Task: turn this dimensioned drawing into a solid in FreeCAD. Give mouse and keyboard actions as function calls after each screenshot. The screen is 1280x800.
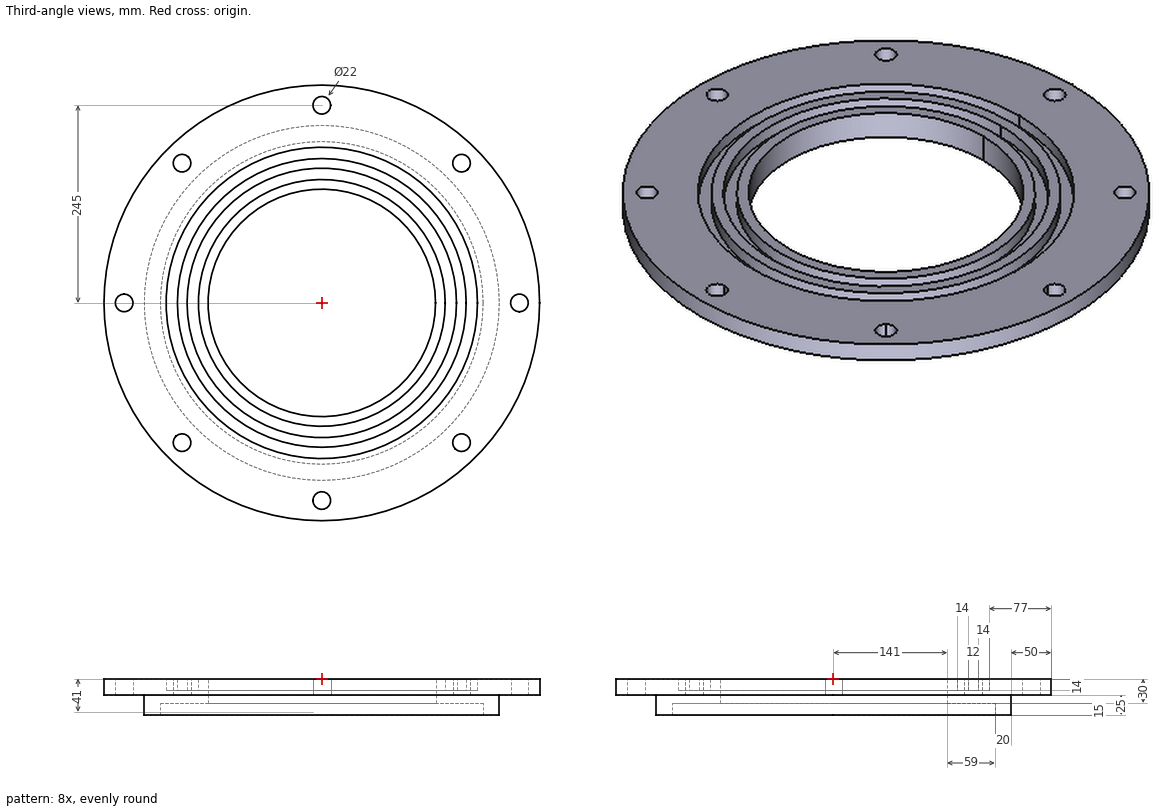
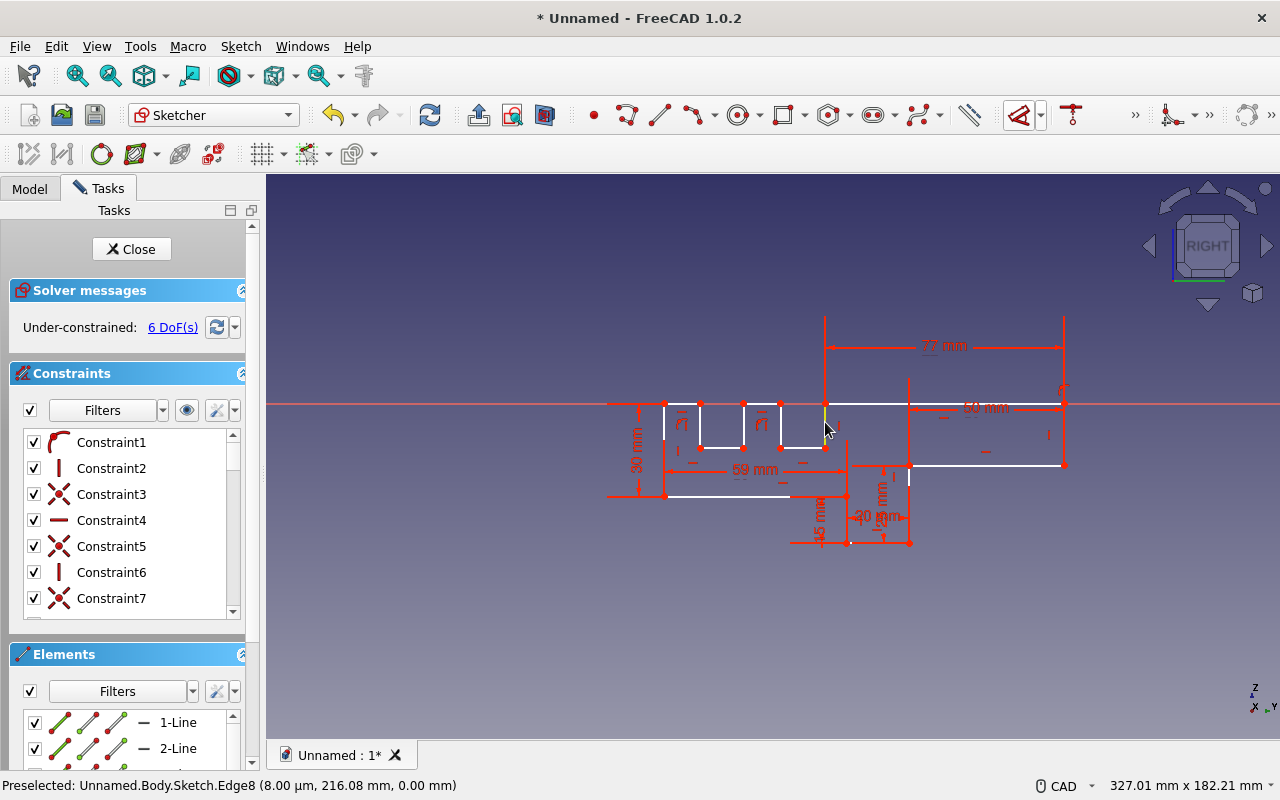
click(825, 422)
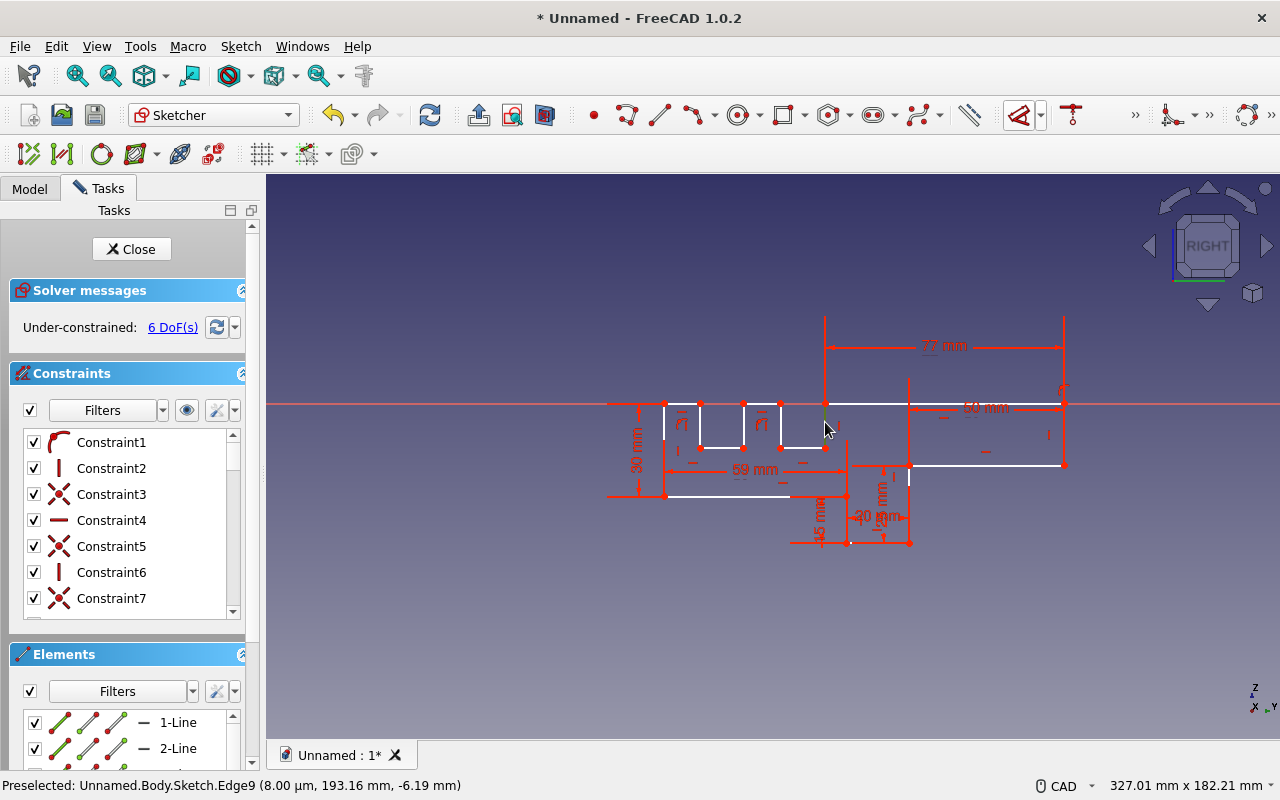
key(i)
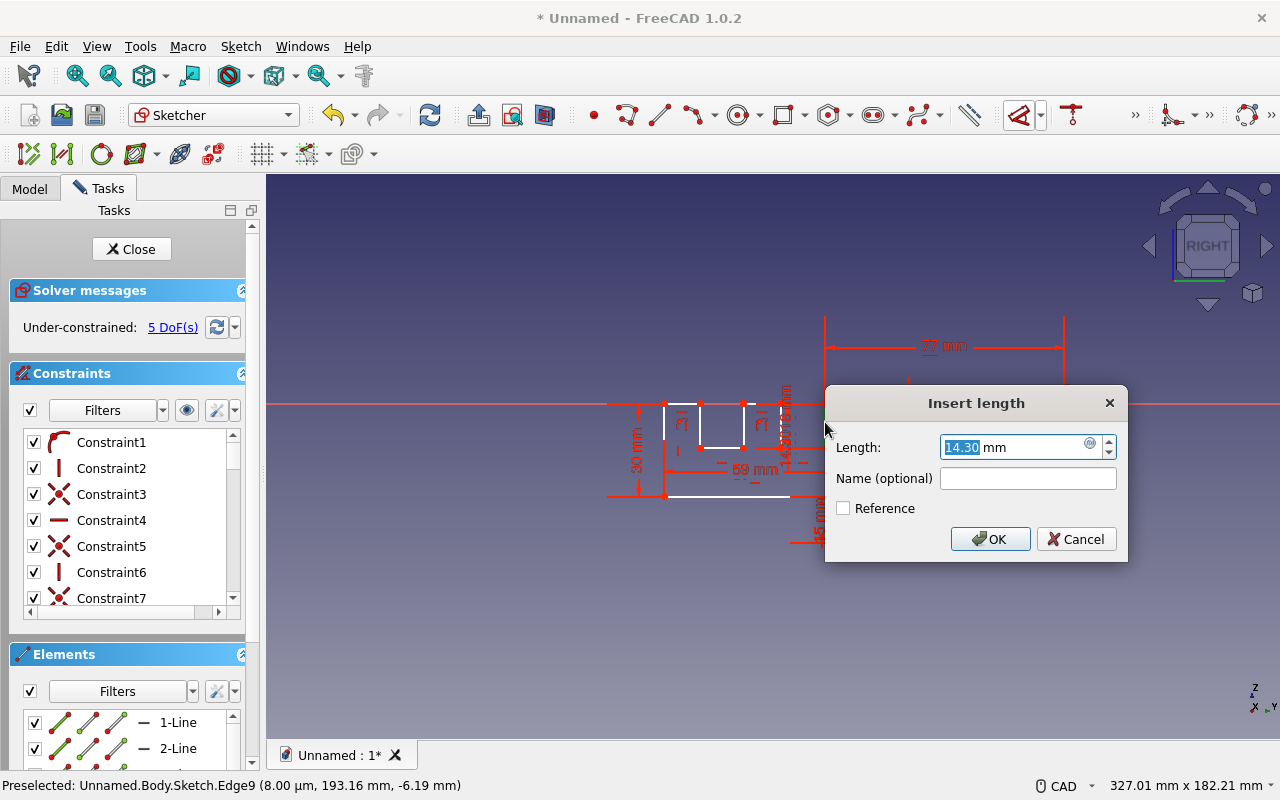
text(14)
key(Return)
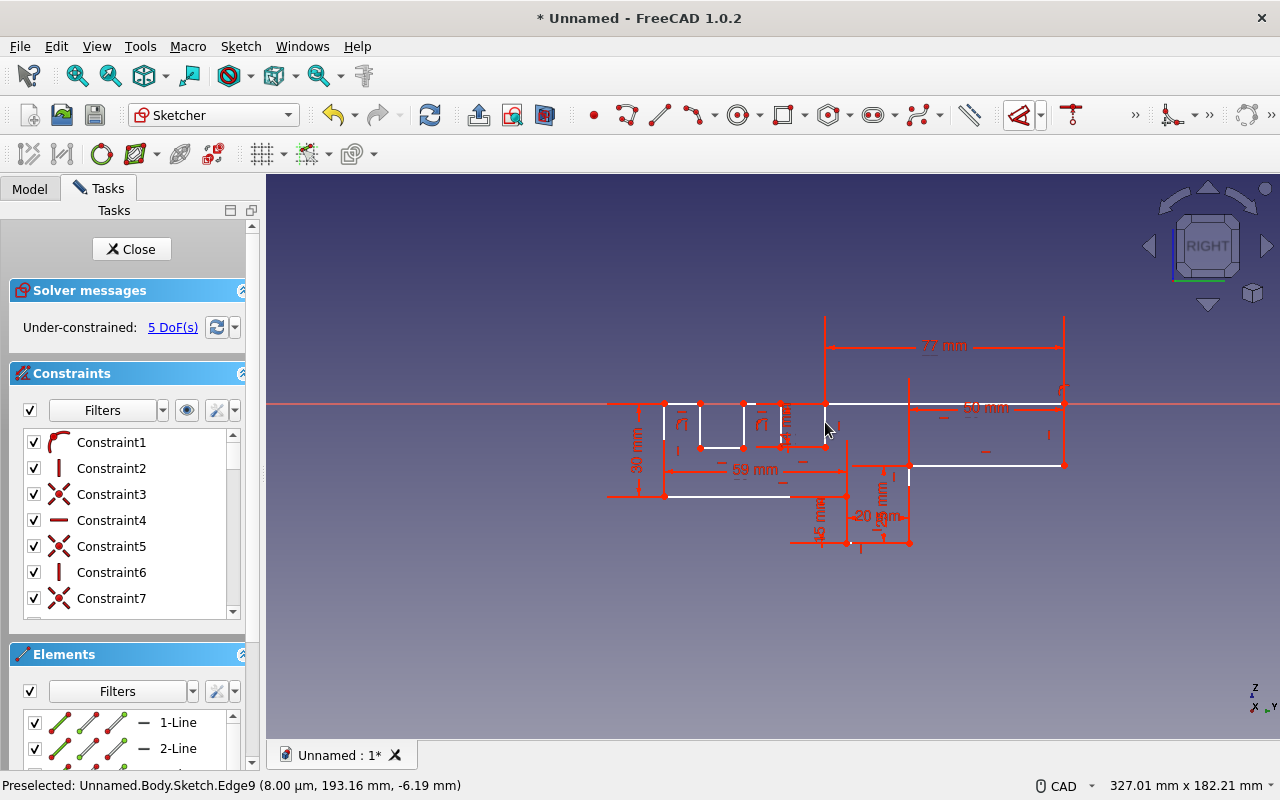
click(812, 447)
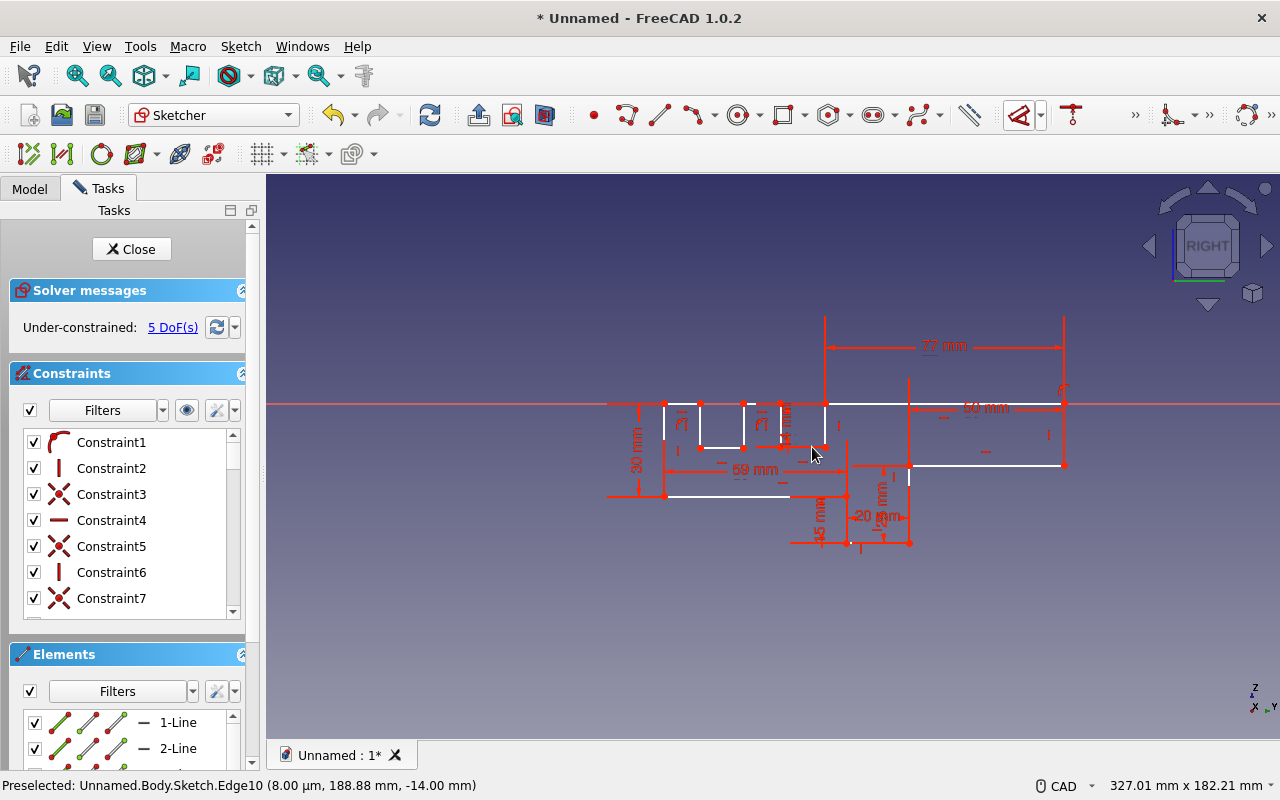
key(l)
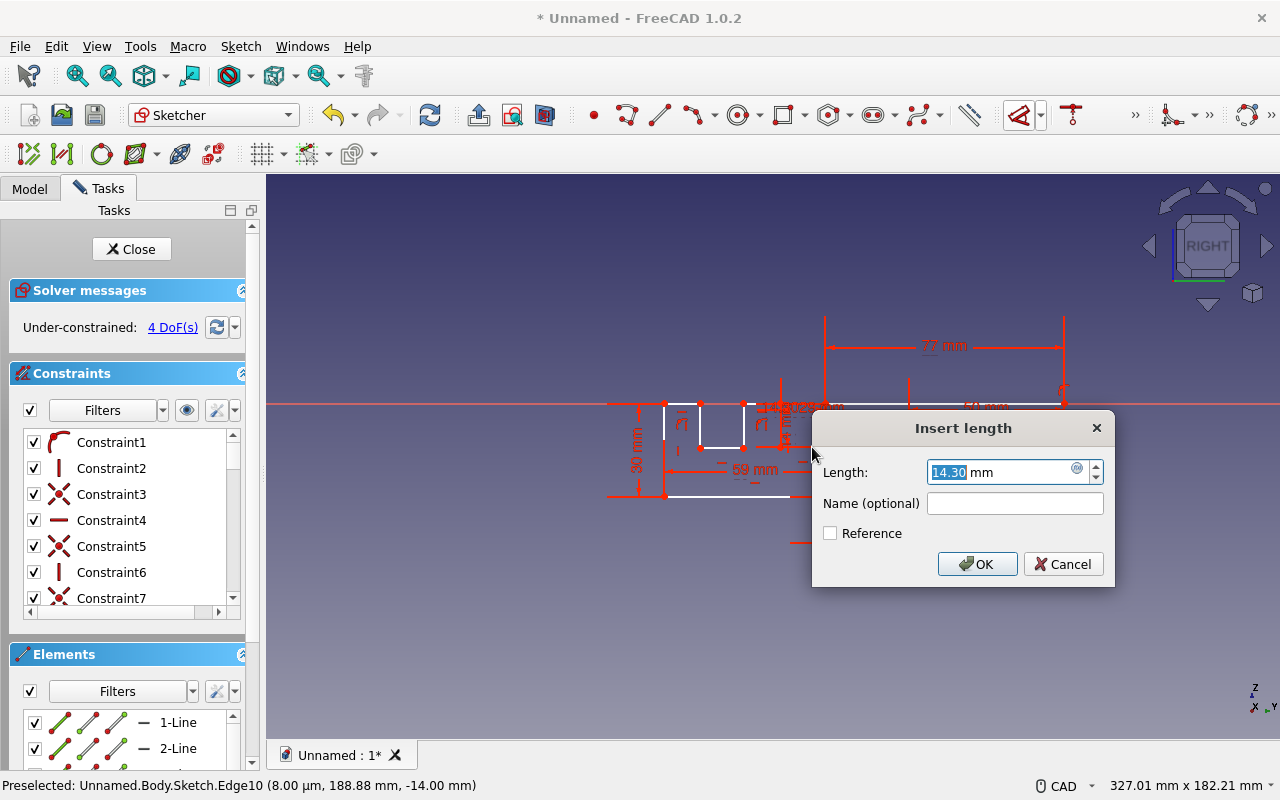
text(14)
key(Return)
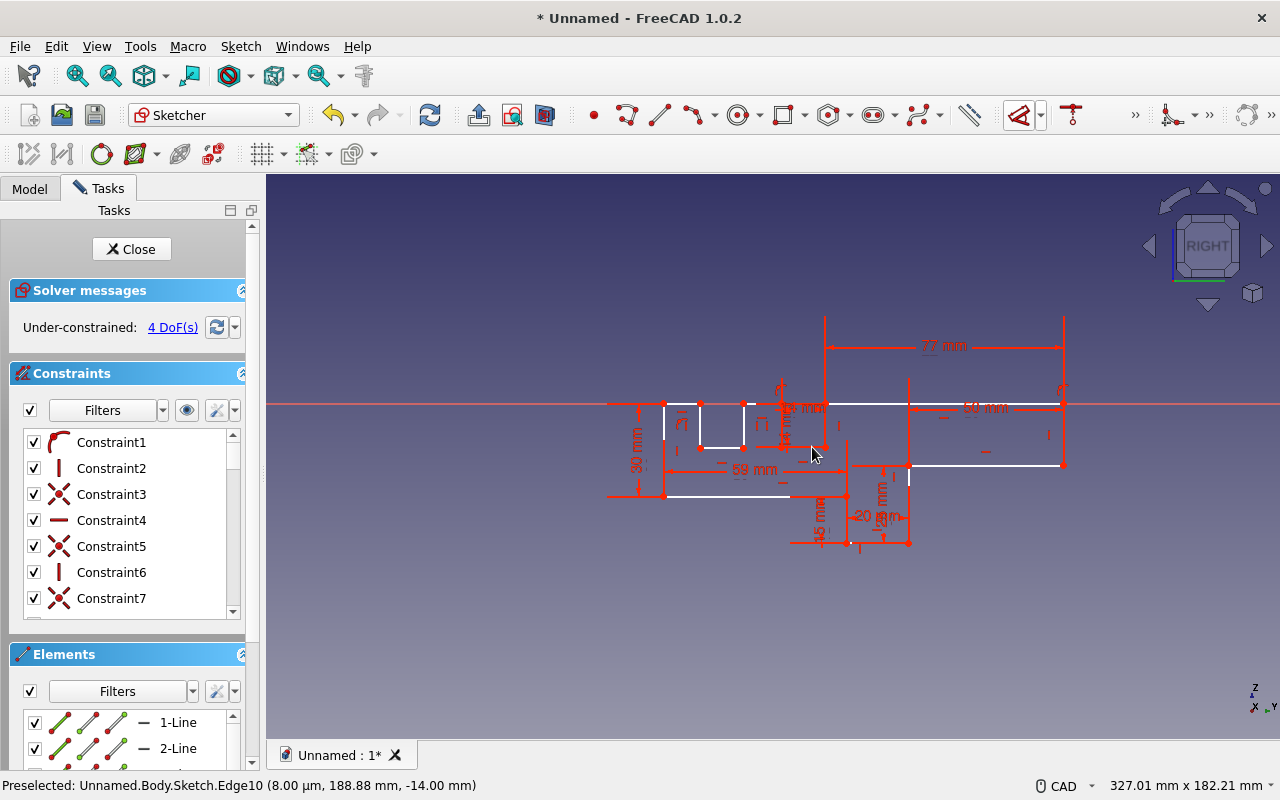
click(770, 404)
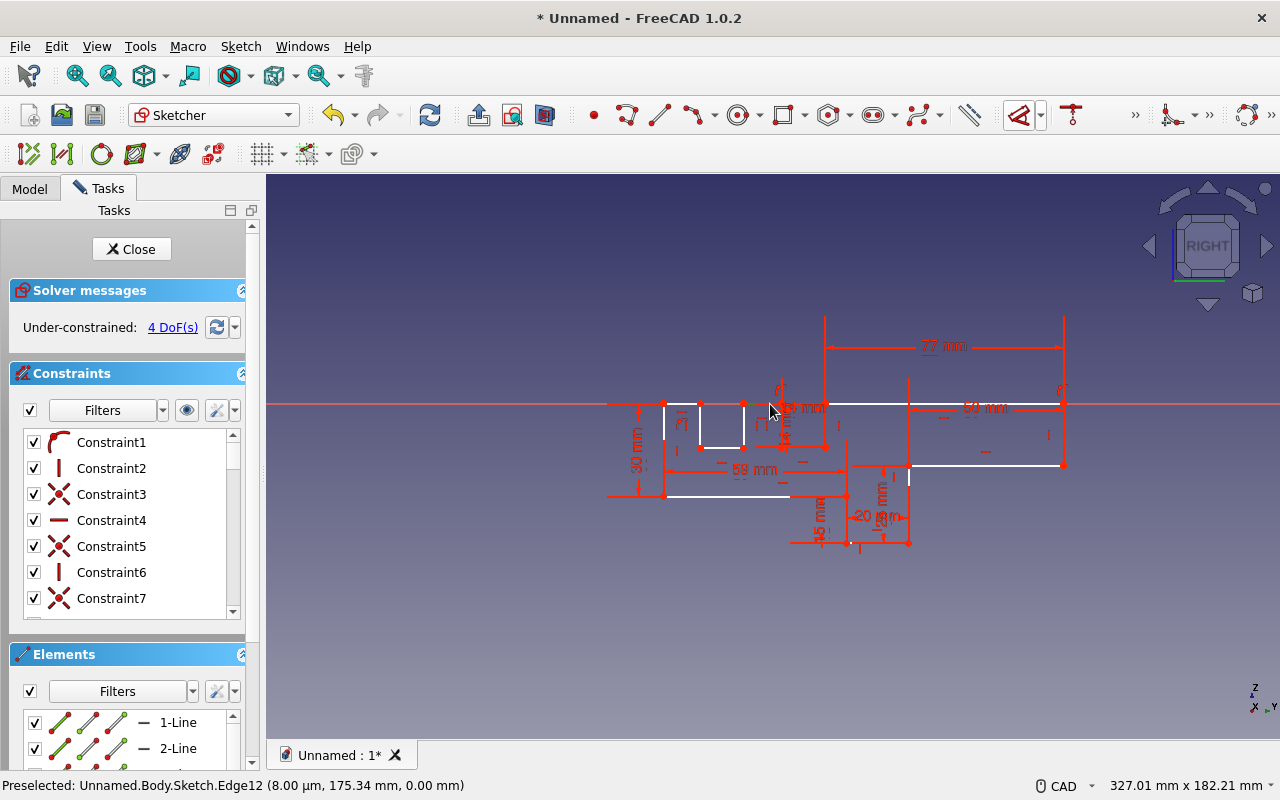
click(1040, 116)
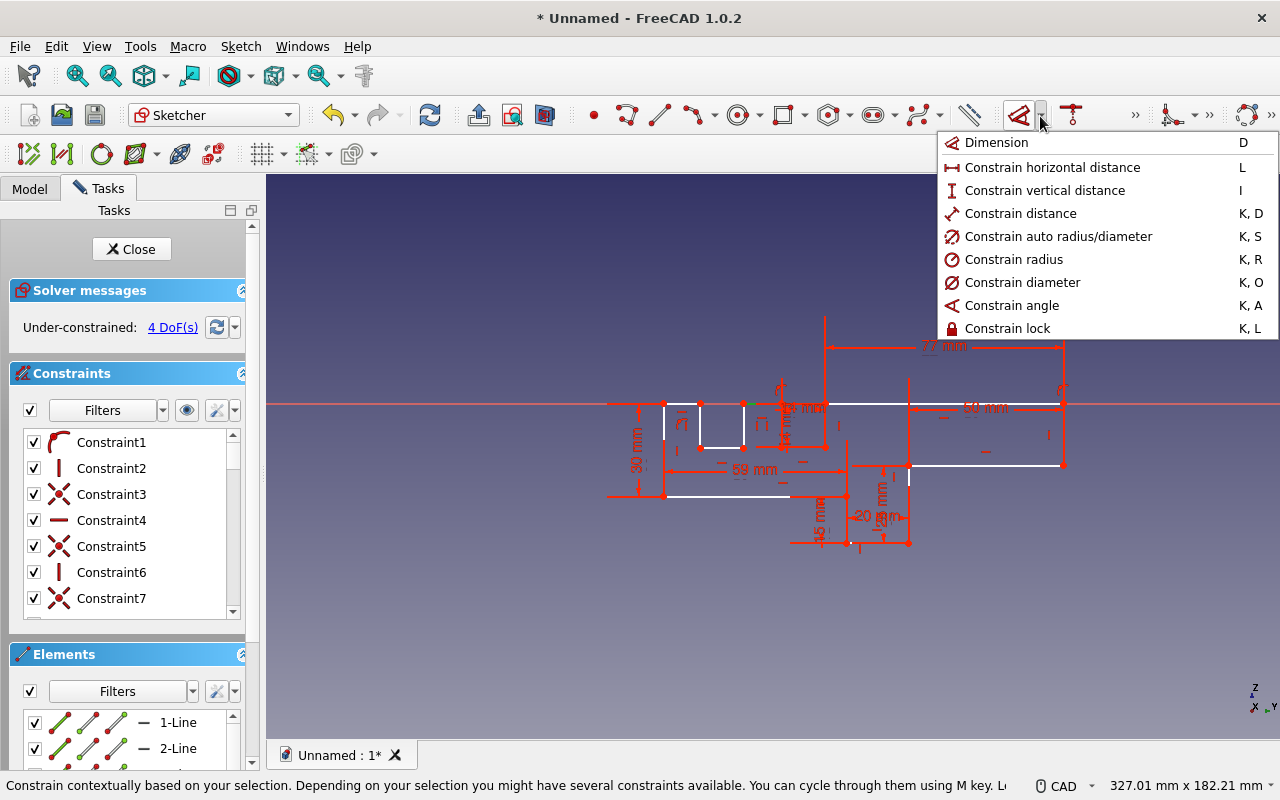
click(1108, 168)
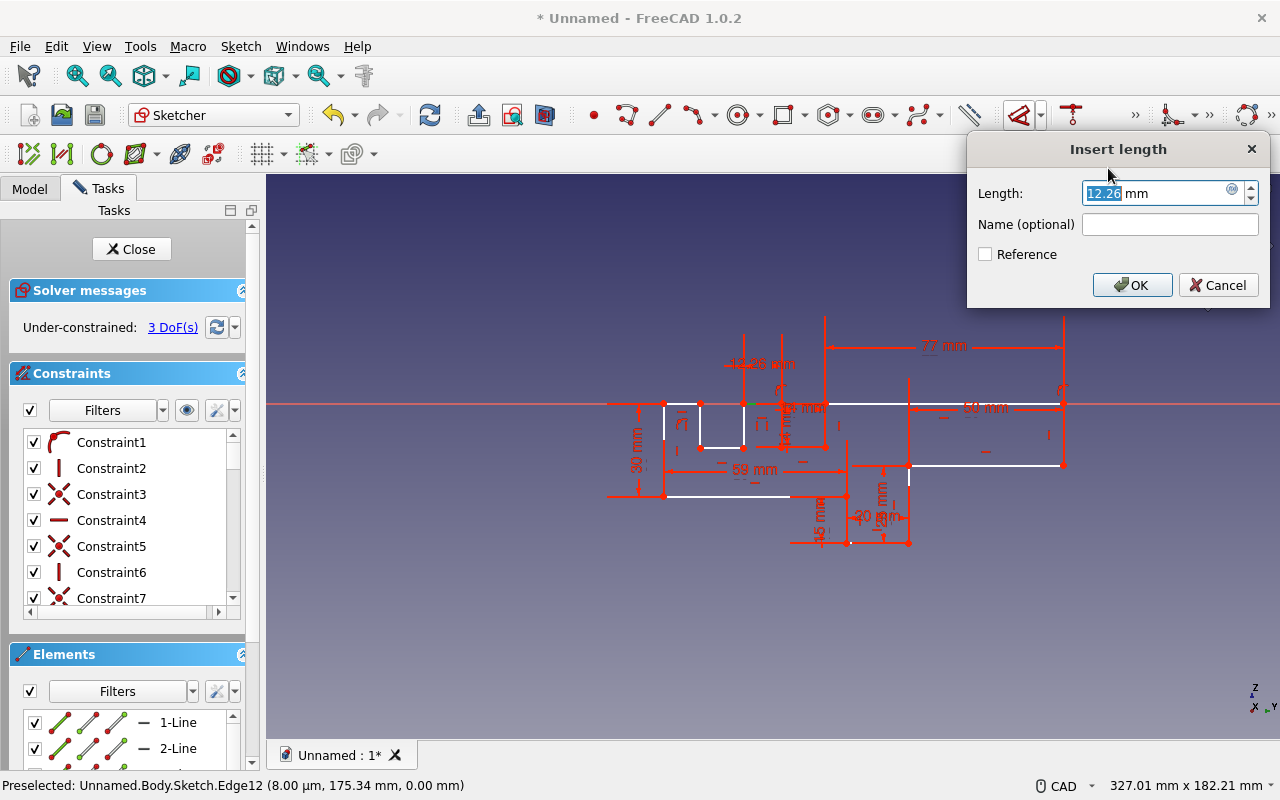
text(12)
key(Return)